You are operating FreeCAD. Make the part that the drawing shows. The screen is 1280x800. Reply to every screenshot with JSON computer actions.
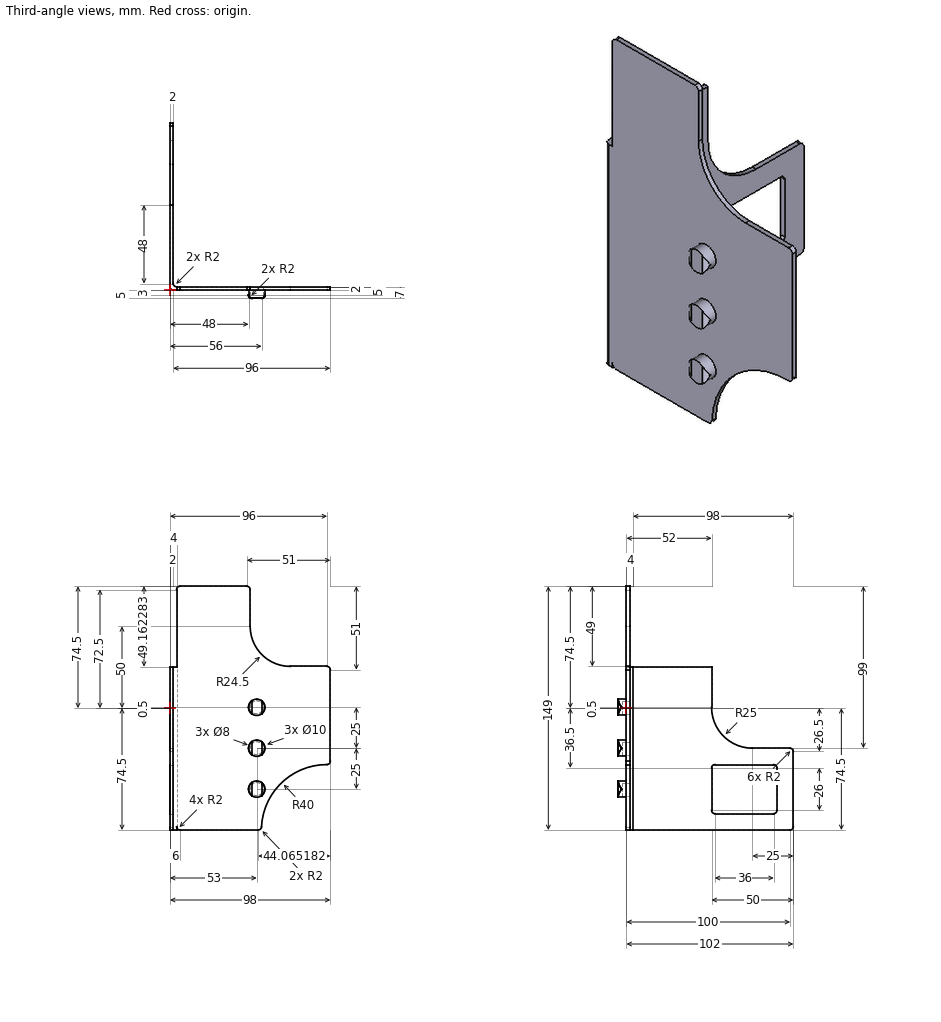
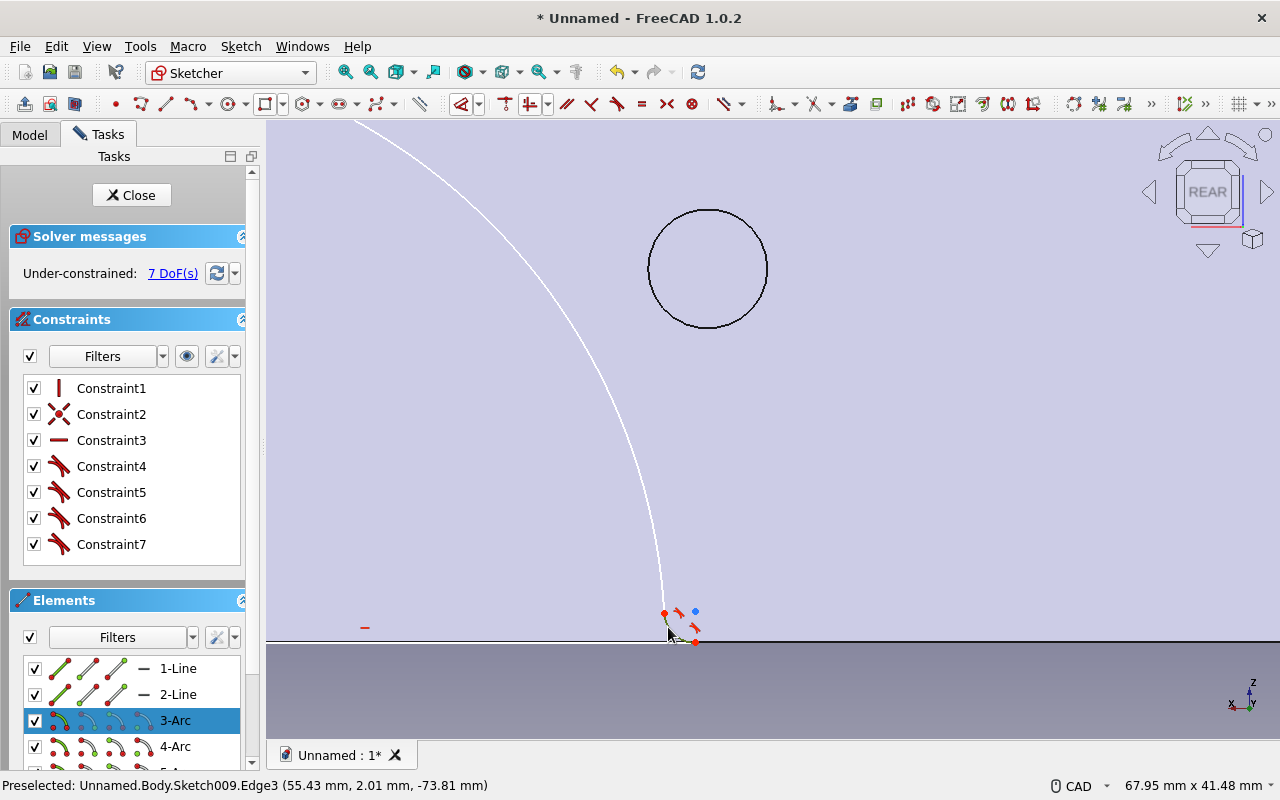
{"action": "scroll", "coordinate": [668, 629], "scroll_direction": "down", "scroll_amount": 5}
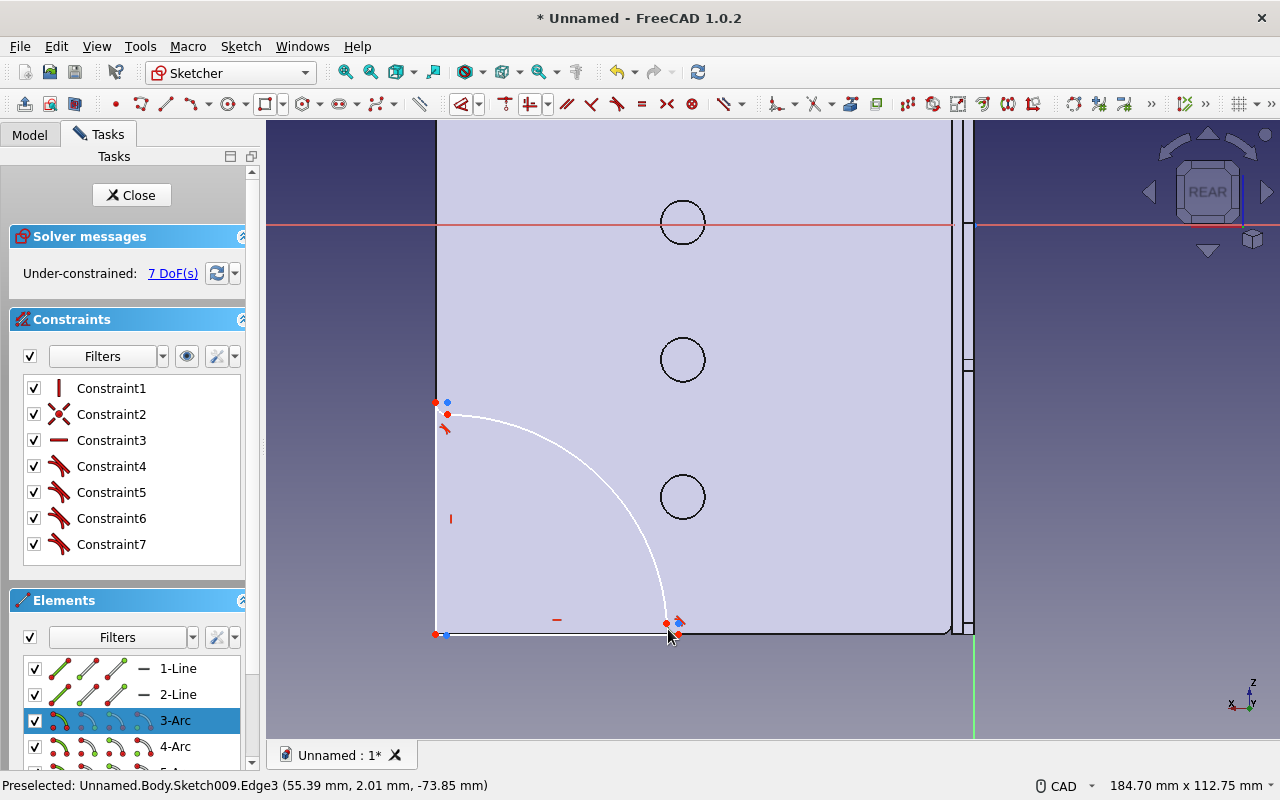
{"action": "scroll", "coordinate": [442, 414], "scroll_direction": "up", "scroll_amount": 5}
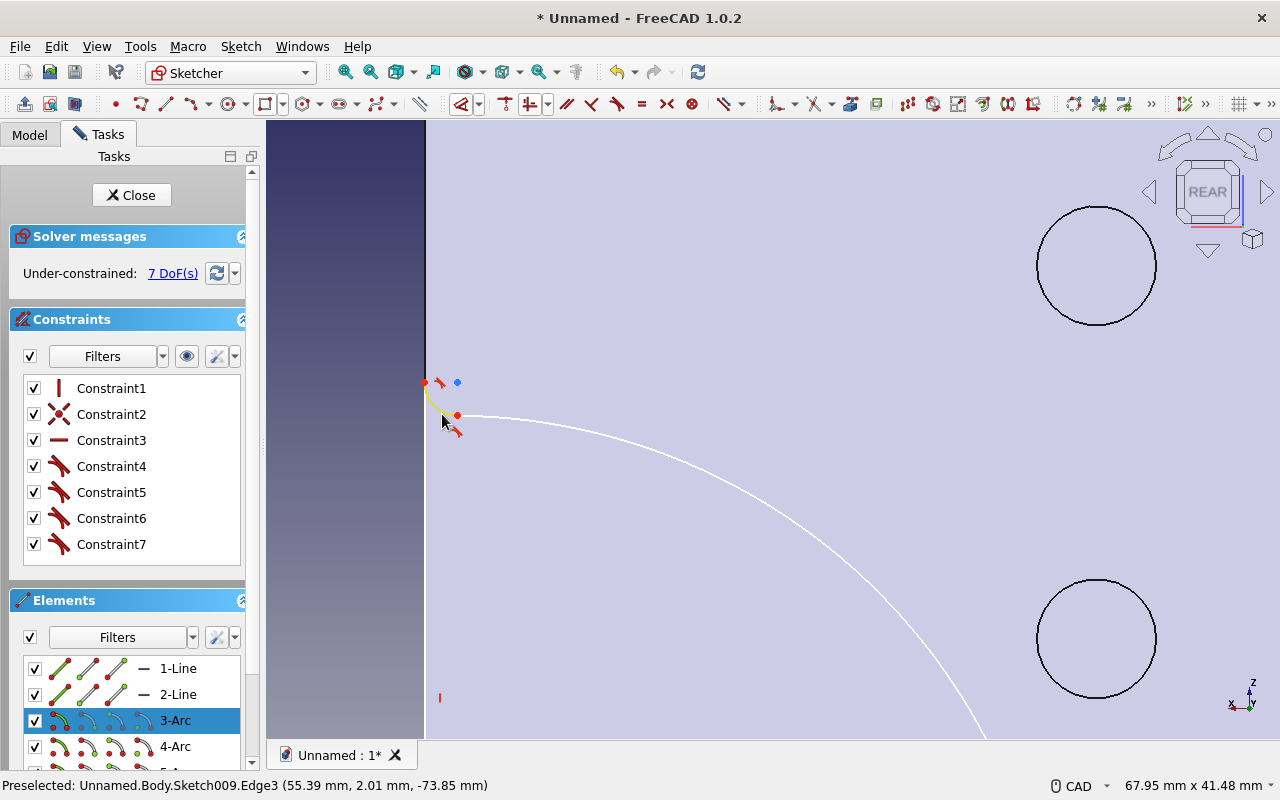
{"action": "left_click", "coordinate": [442, 412]}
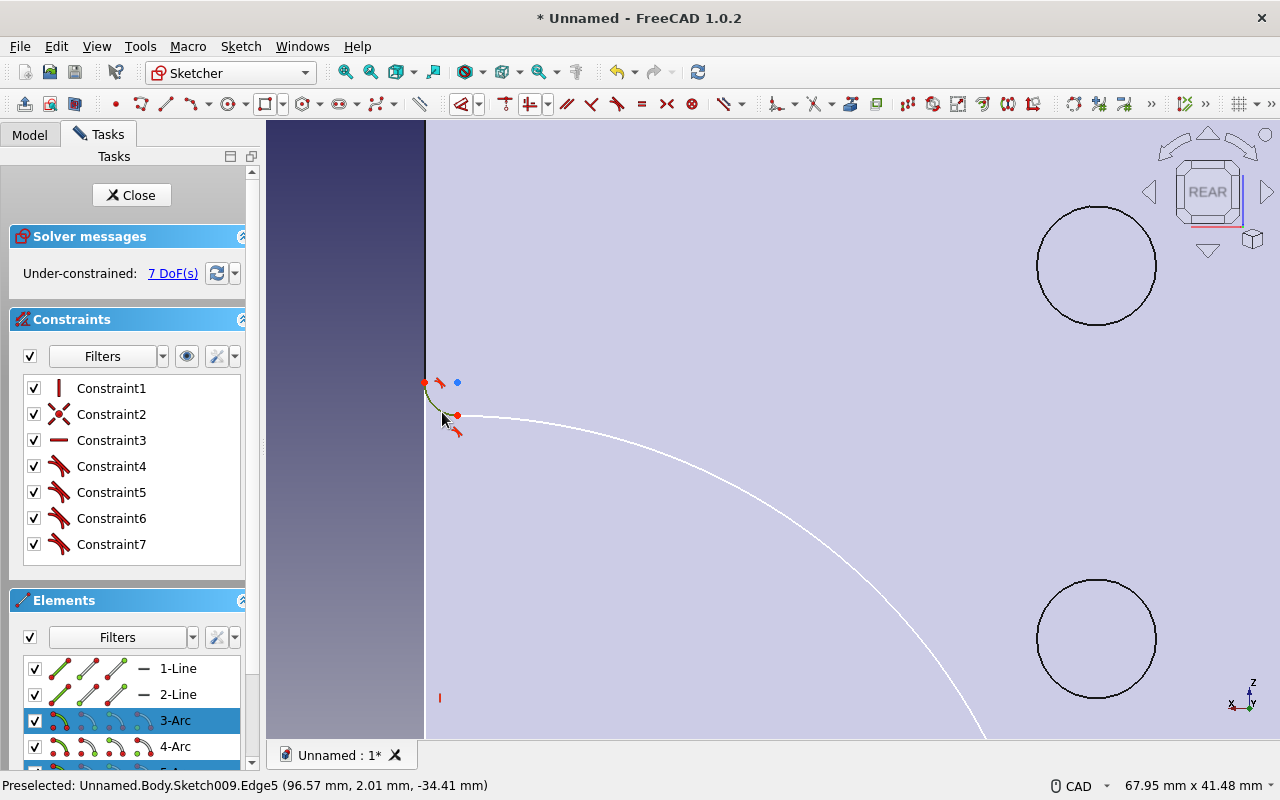
{"action": "key", "text": "e"}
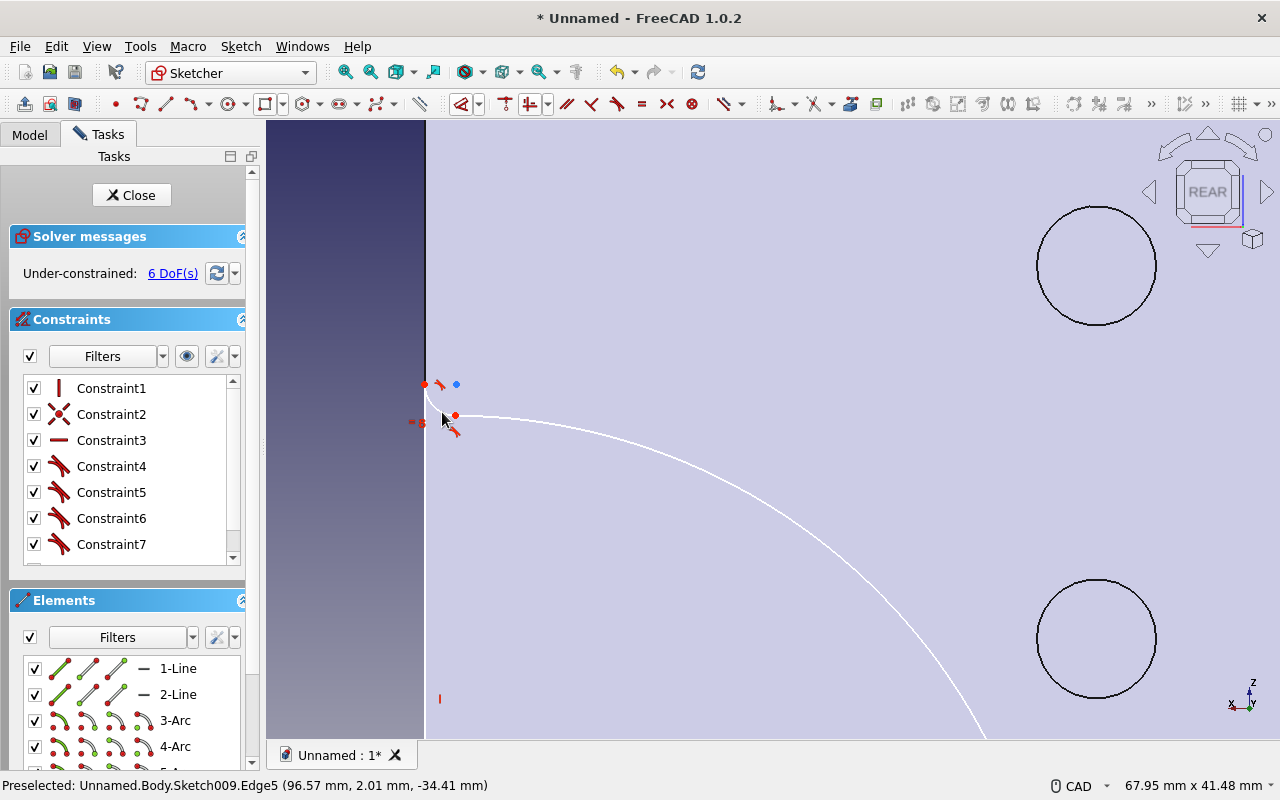
{"action": "scroll", "coordinate": [442, 414], "scroll_direction": "down", "scroll_amount": 5}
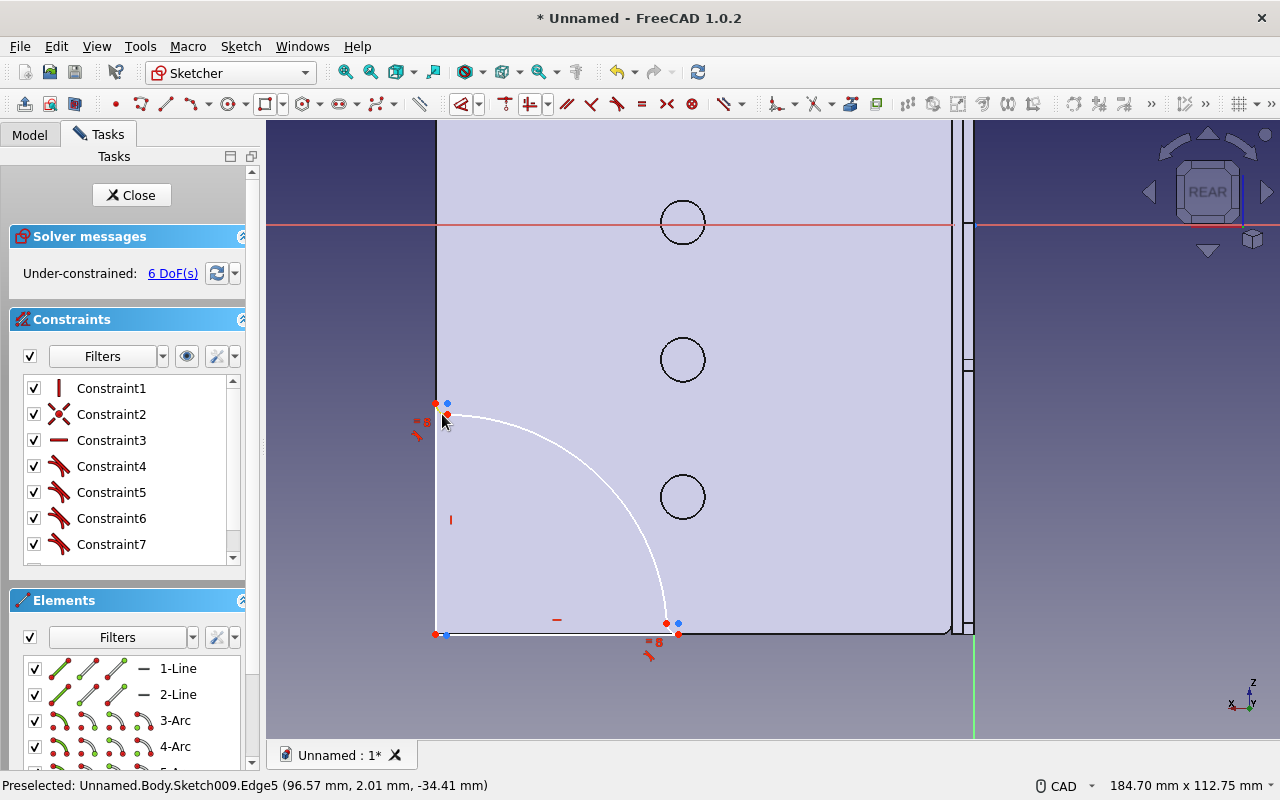
{"action": "scroll", "coordinate": [668, 629], "scroll_direction": "up", "scroll_amount": 7}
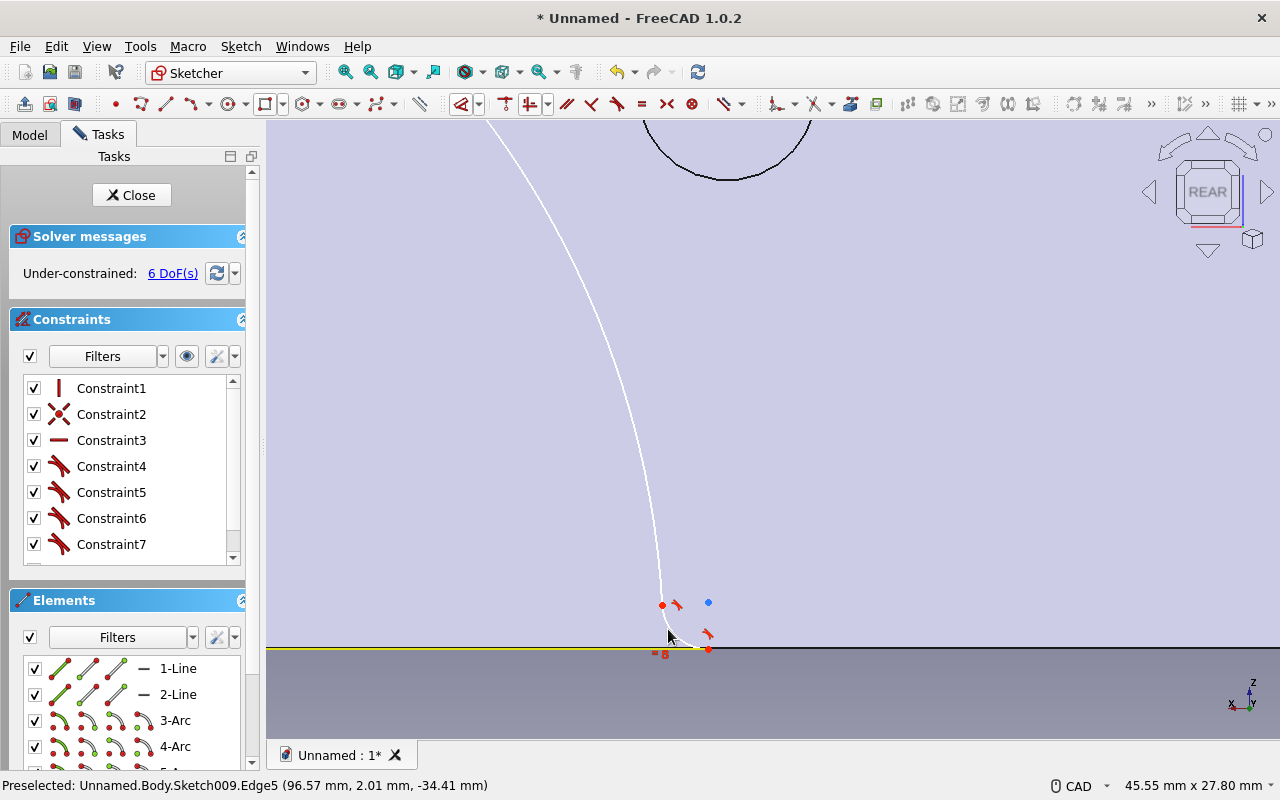
{"action": "left_click", "coordinate": [668, 625]}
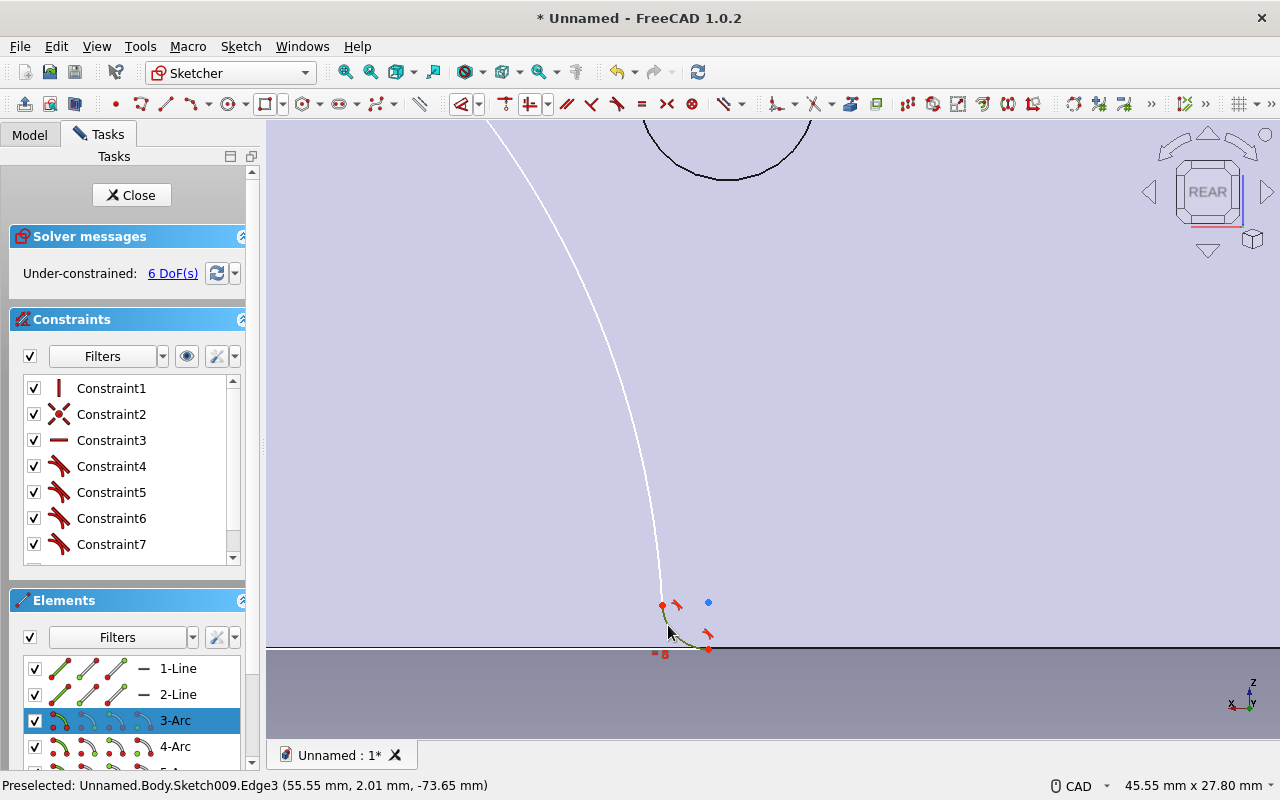
{"action": "key", "text": "k r"}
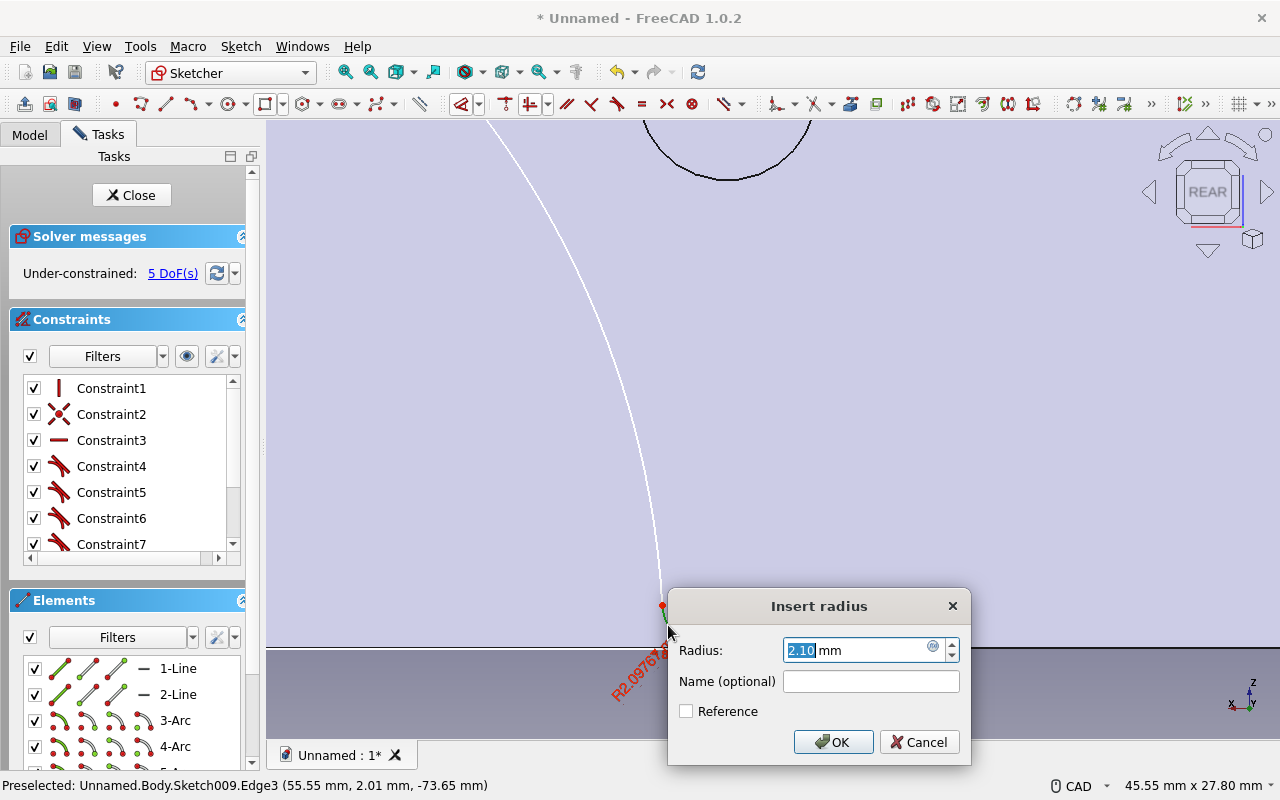
{"action": "type", "text": "2"}
{"action": "key", "text": "Return"}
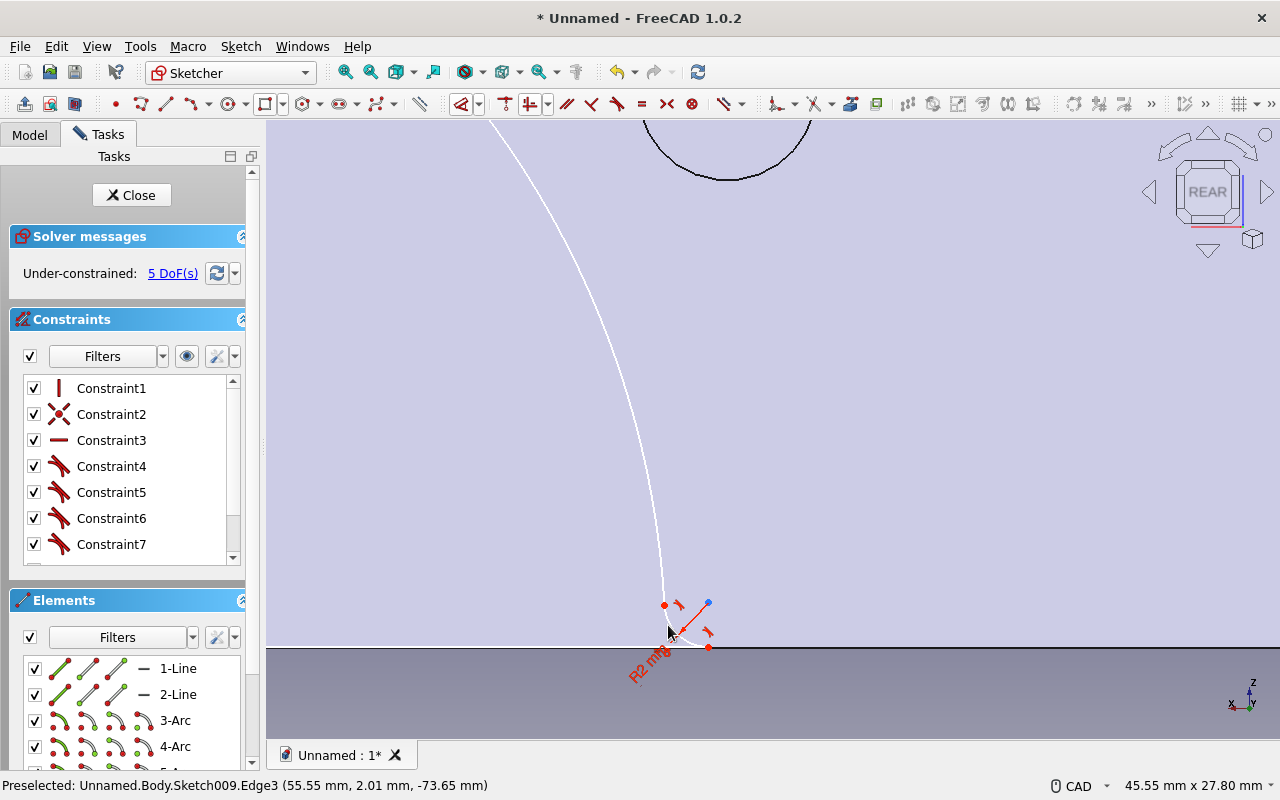
{"action": "scroll", "coordinate": [668, 629], "scroll_direction": "down", "scroll_amount": 7}